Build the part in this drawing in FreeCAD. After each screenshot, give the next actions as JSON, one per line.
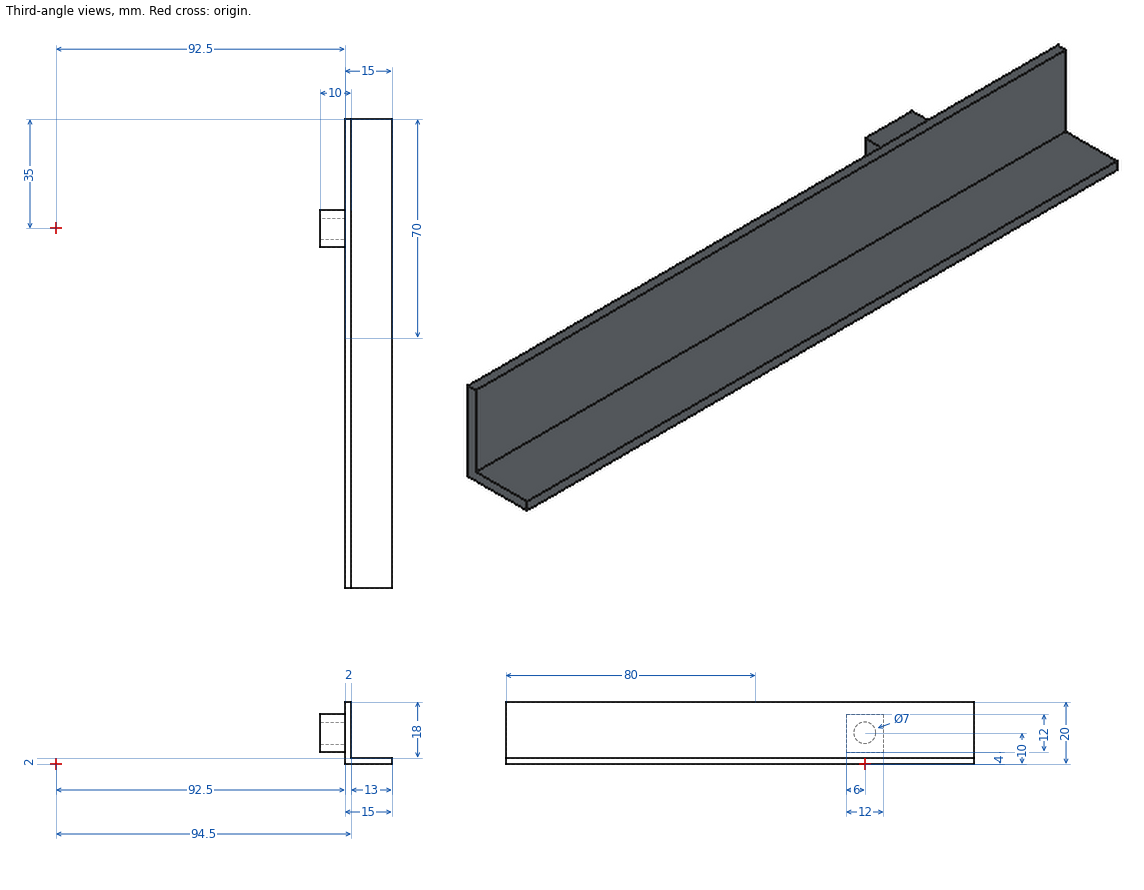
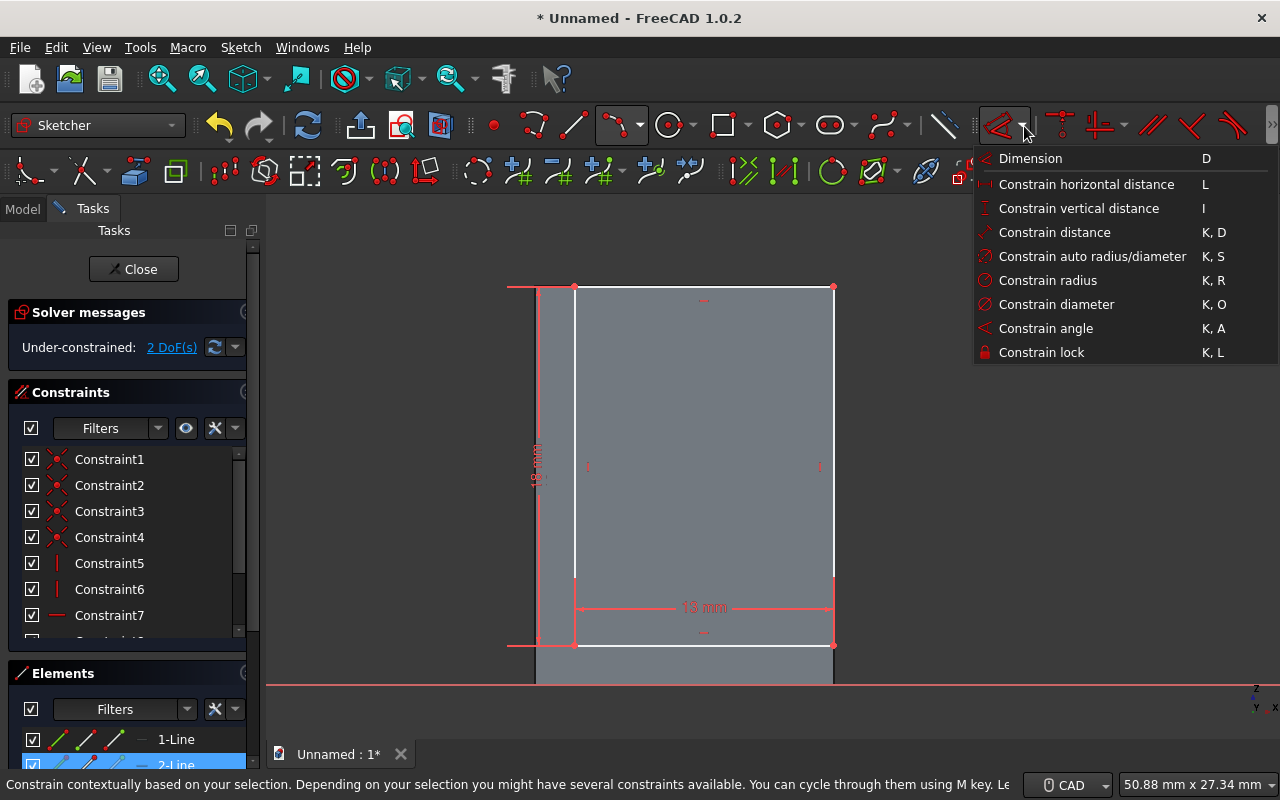
{"action": "left_click", "coordinate": [1126, 208]}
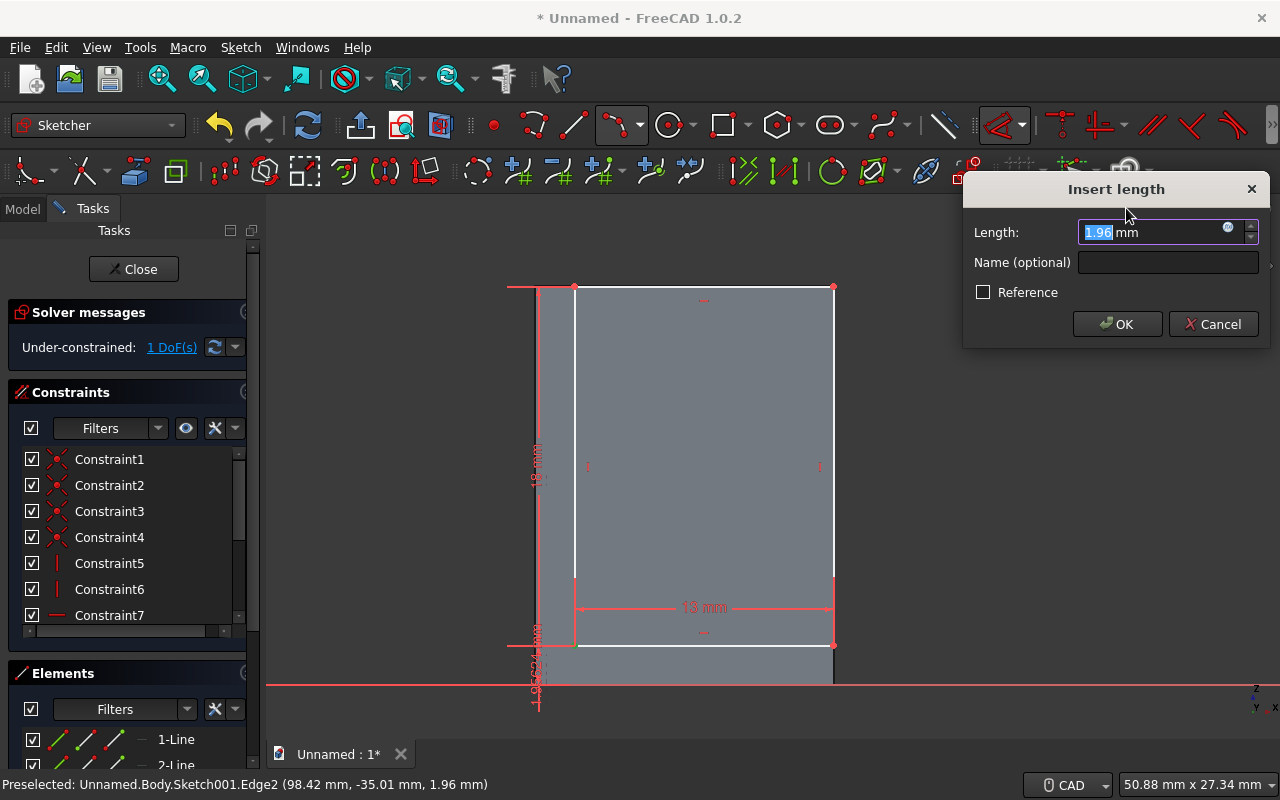
{"action": "type", "text": "2"}
{"action": "key", "text": "Return"}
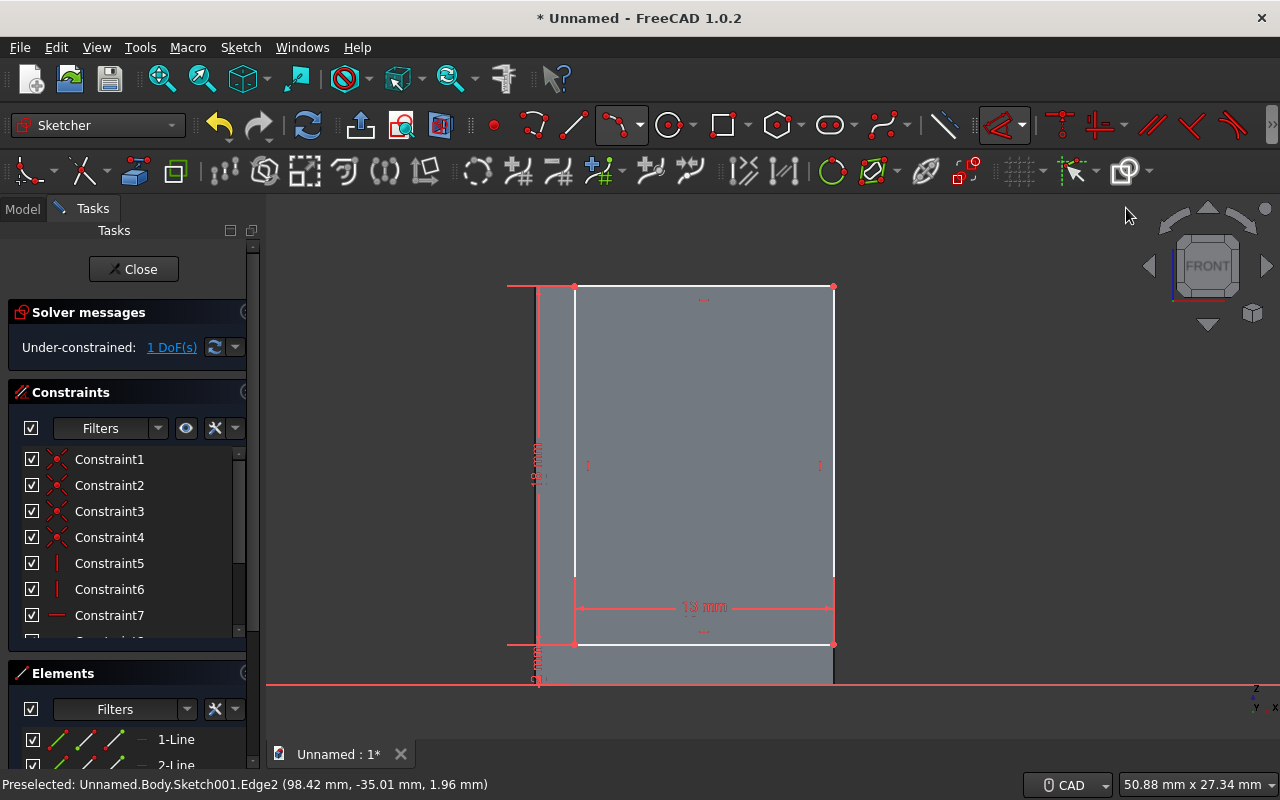
{"action": "left_click", "coordinate": [575, 286]}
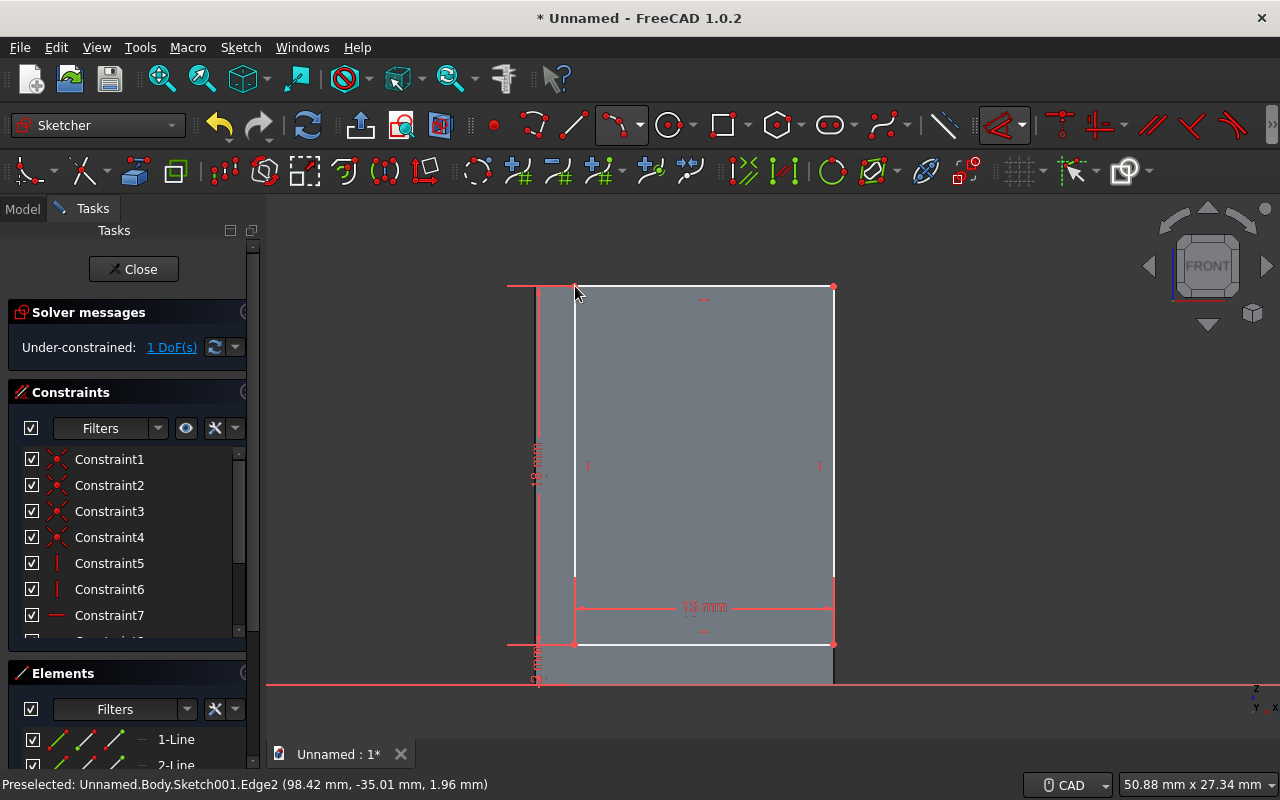
{"action": "left_click", "coordinate": [1024, 126]}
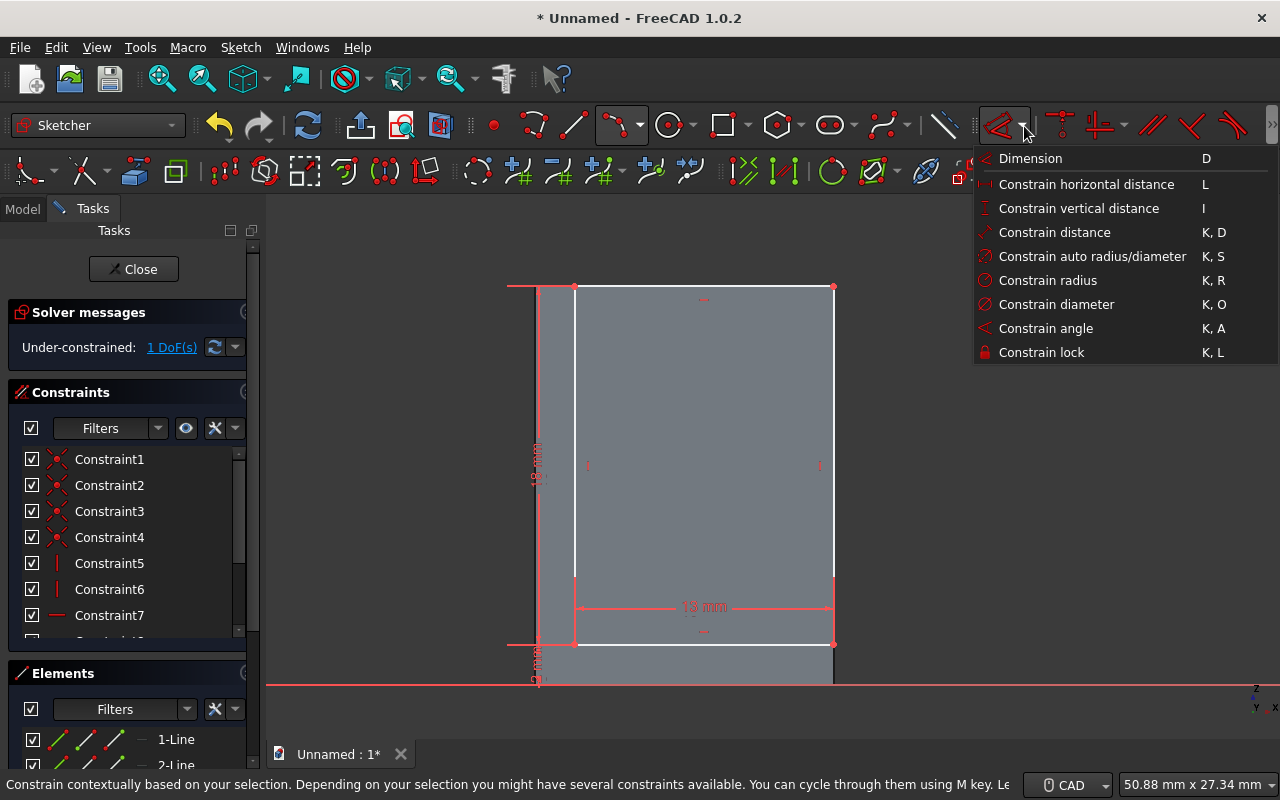
{"action": "left_click", "coordinate": [1126, 184]}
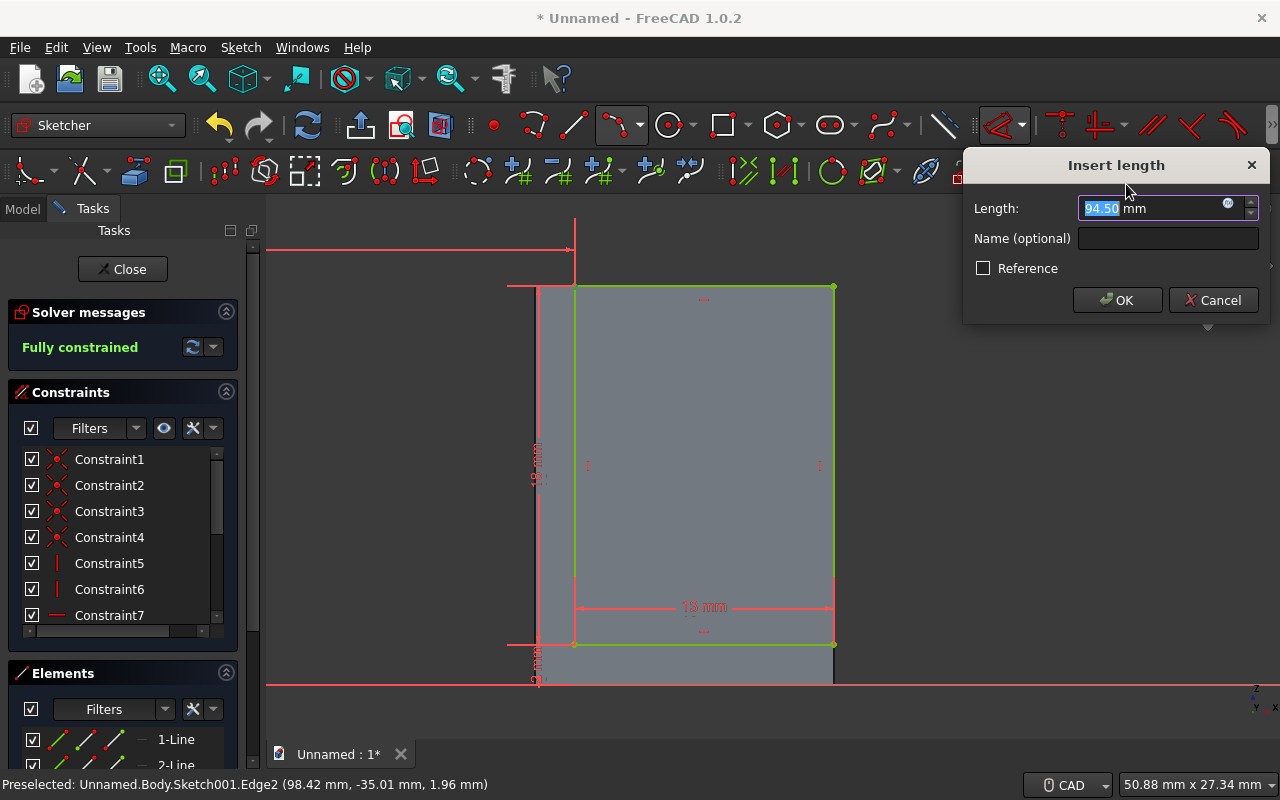
{"action": "type", "text": "94.5"}
{"action": "key", "text": "Return"}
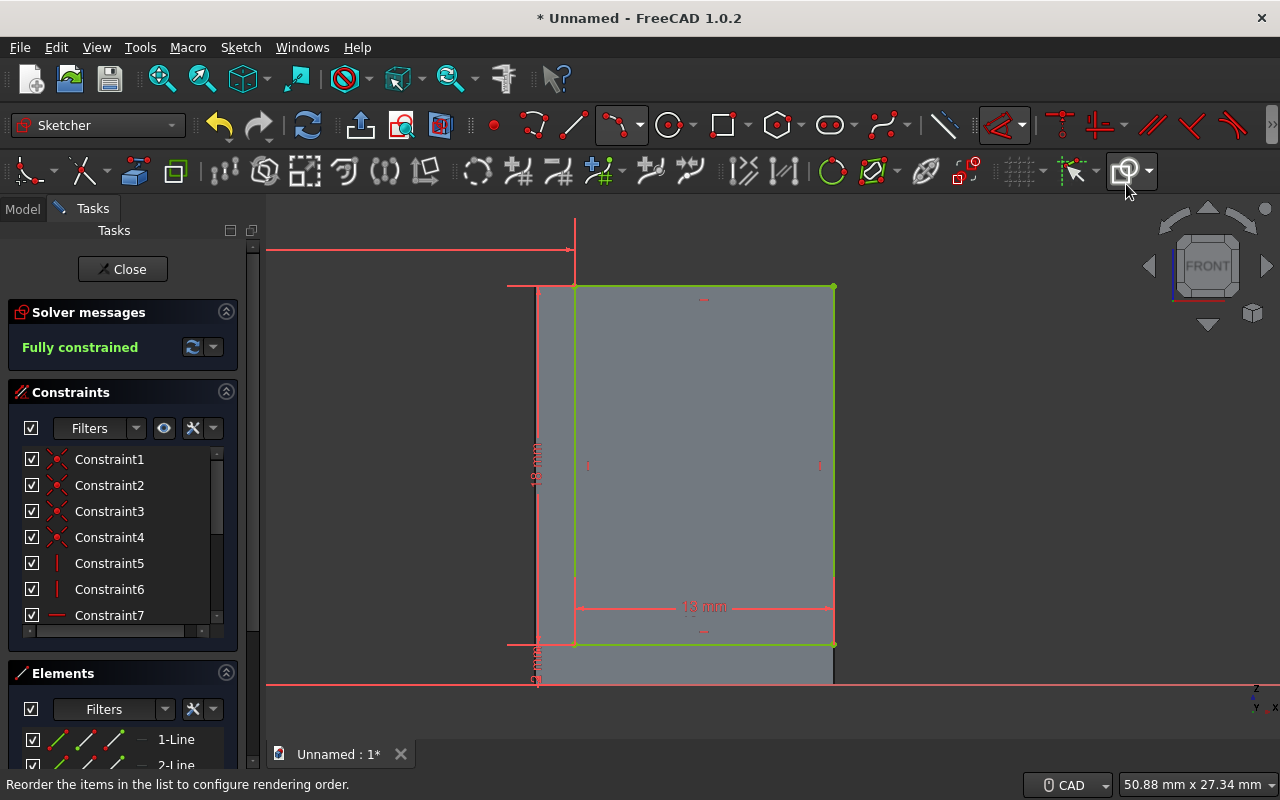
{"action": "left_click", "coordinate": [123, 269]}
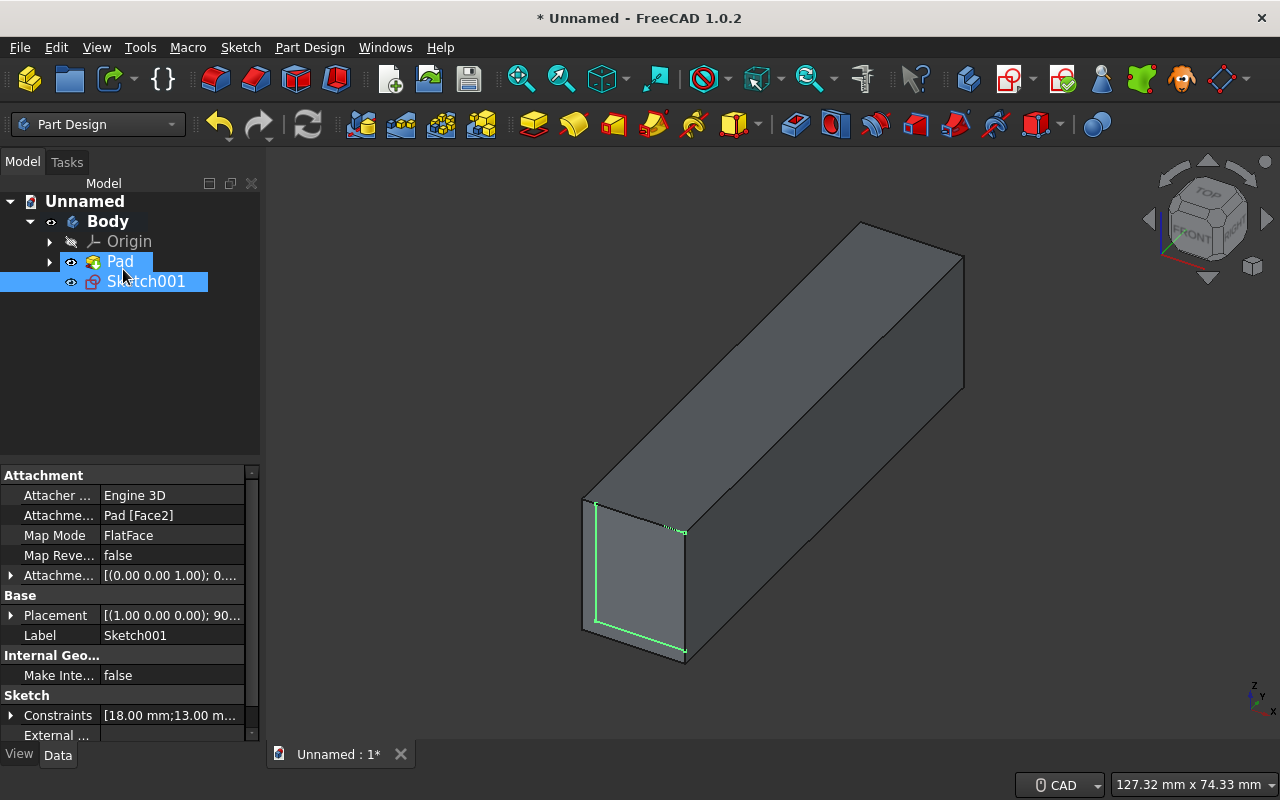
{"action": "left_click", "coordinate": [796, 124]}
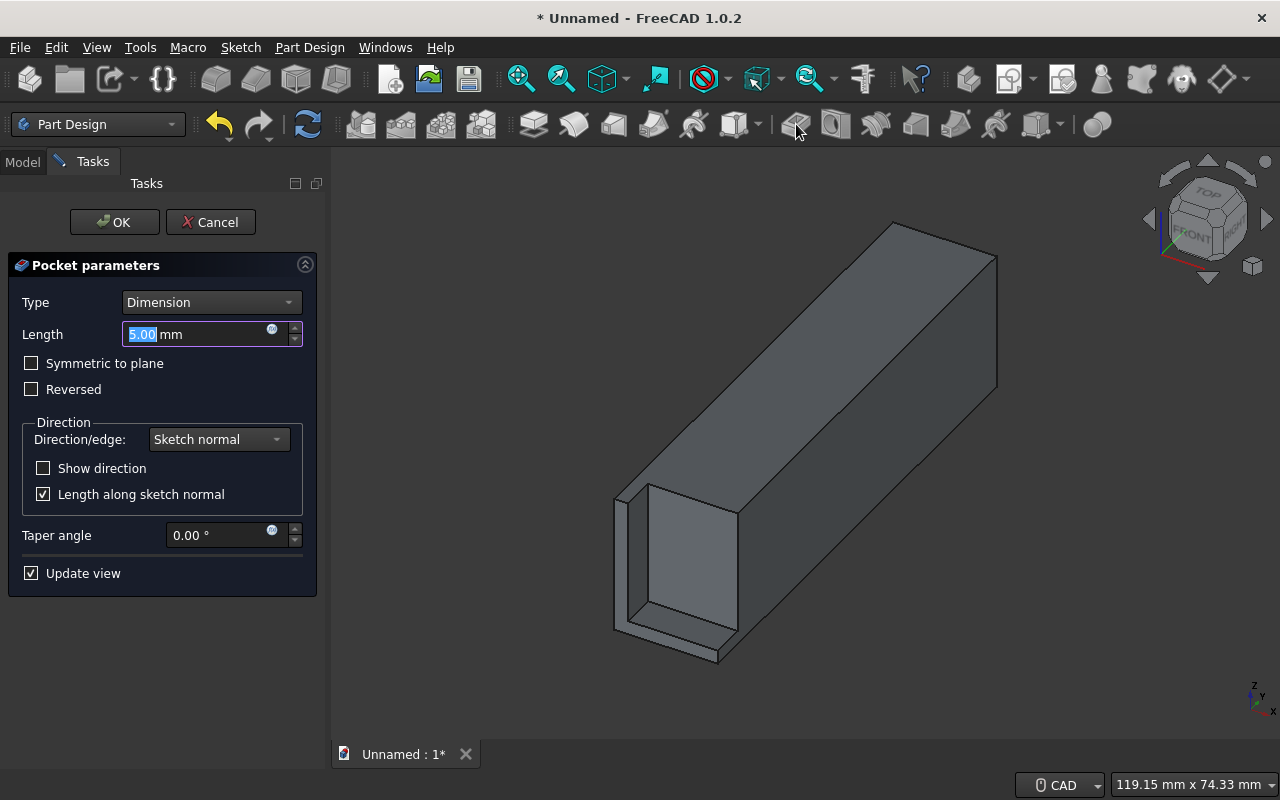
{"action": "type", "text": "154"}
{"action": "key", "text": "Tab"}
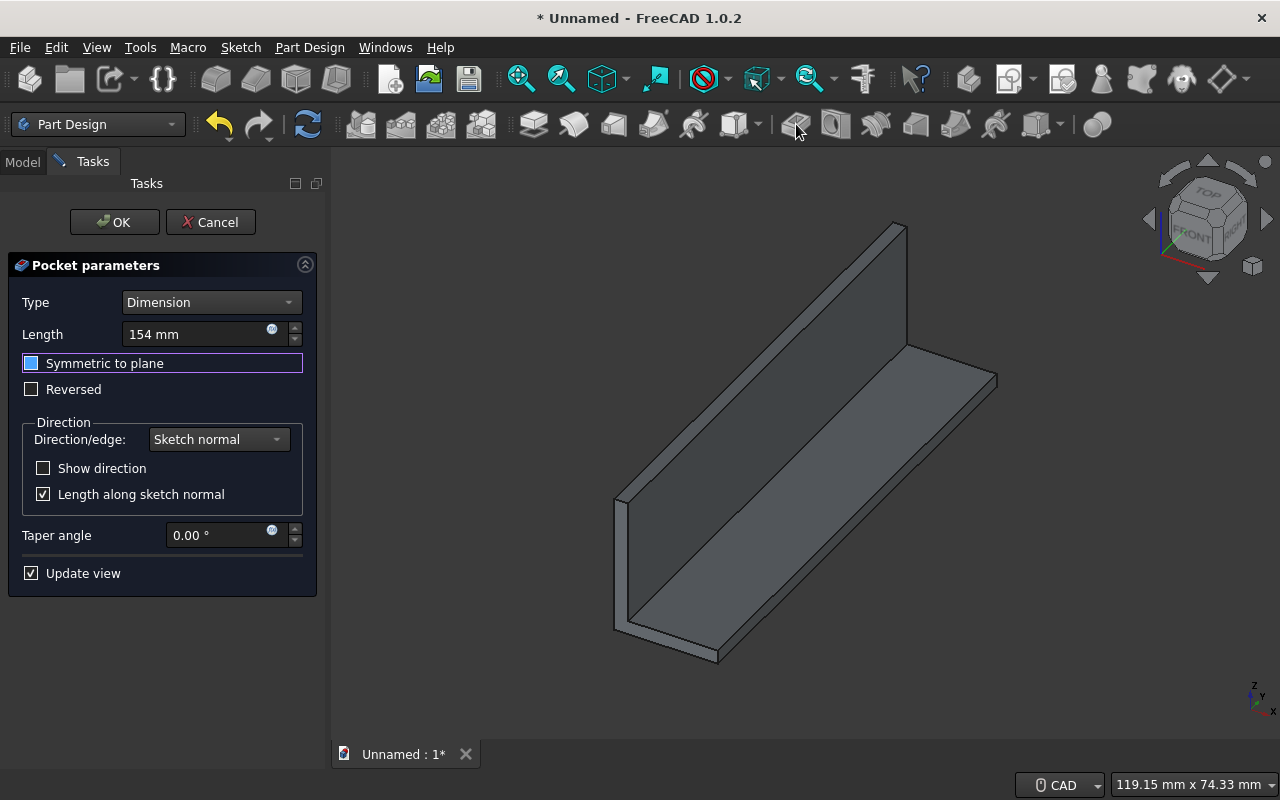
{"action": "left_click", "coordinate": [115, 222]}